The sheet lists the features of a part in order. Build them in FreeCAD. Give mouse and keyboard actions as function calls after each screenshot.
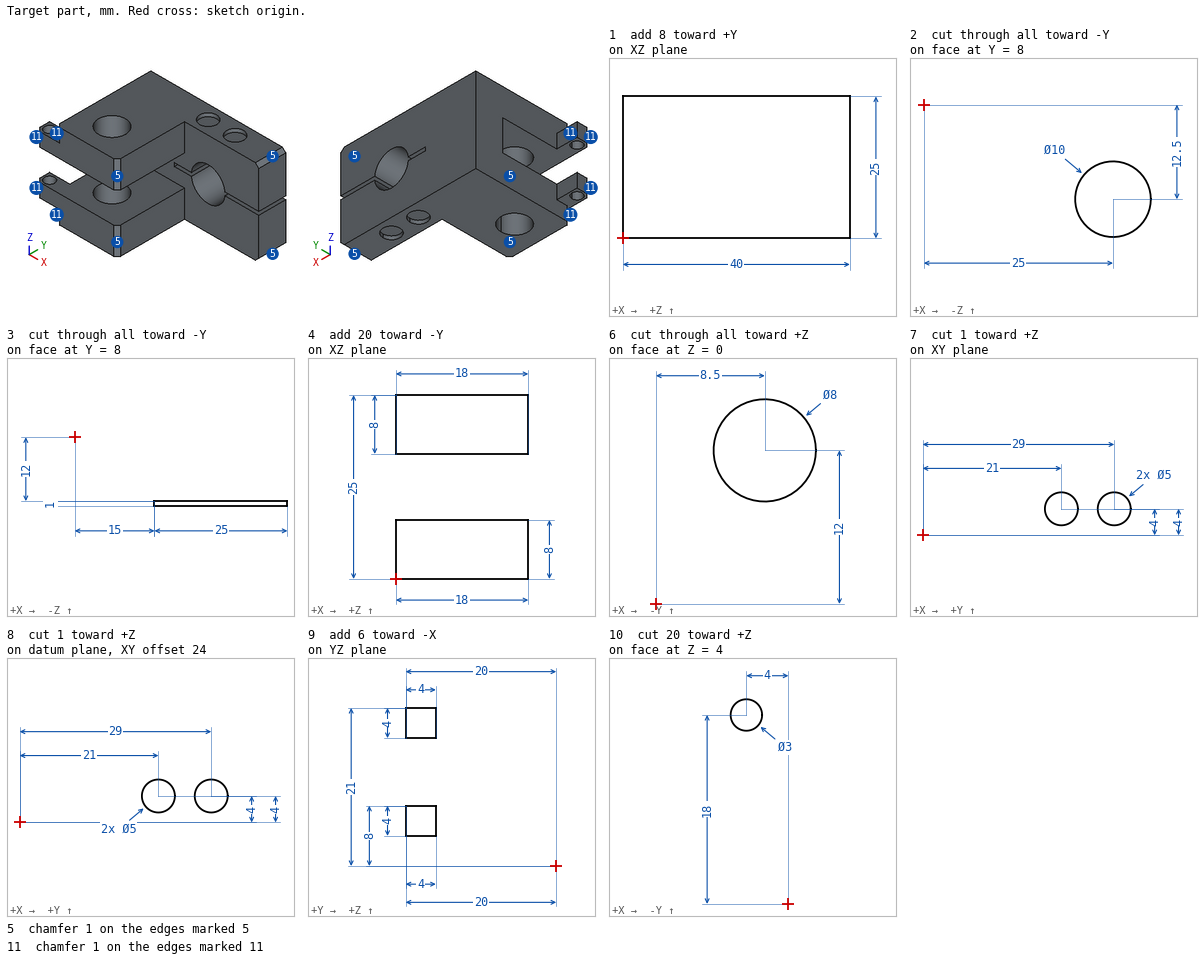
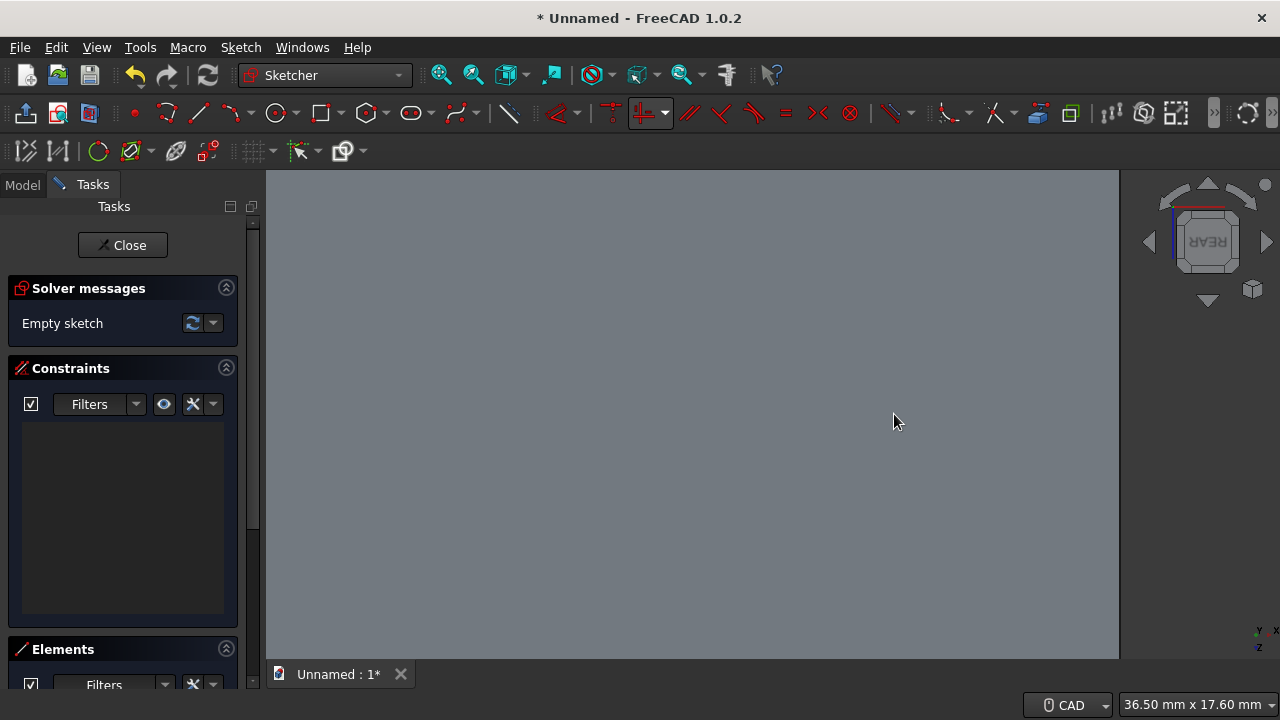
click(276, 114)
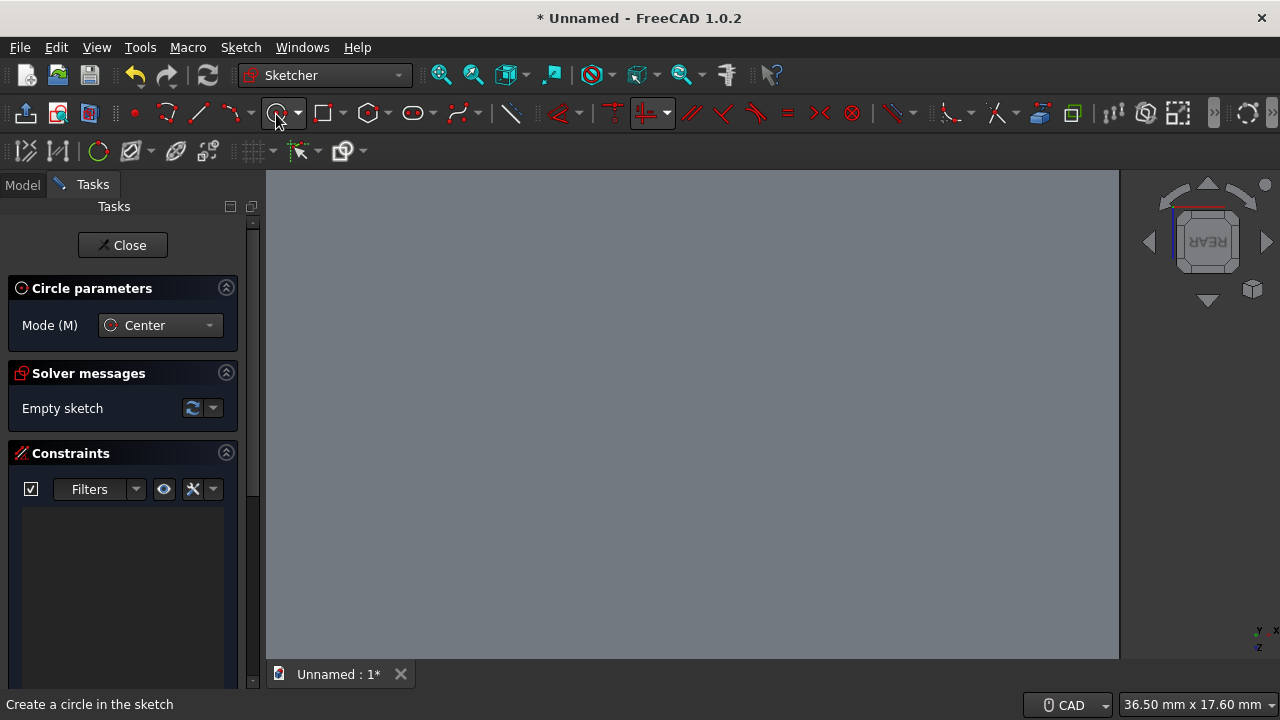
click(703, 414)
click(801, 316)
key(Escape)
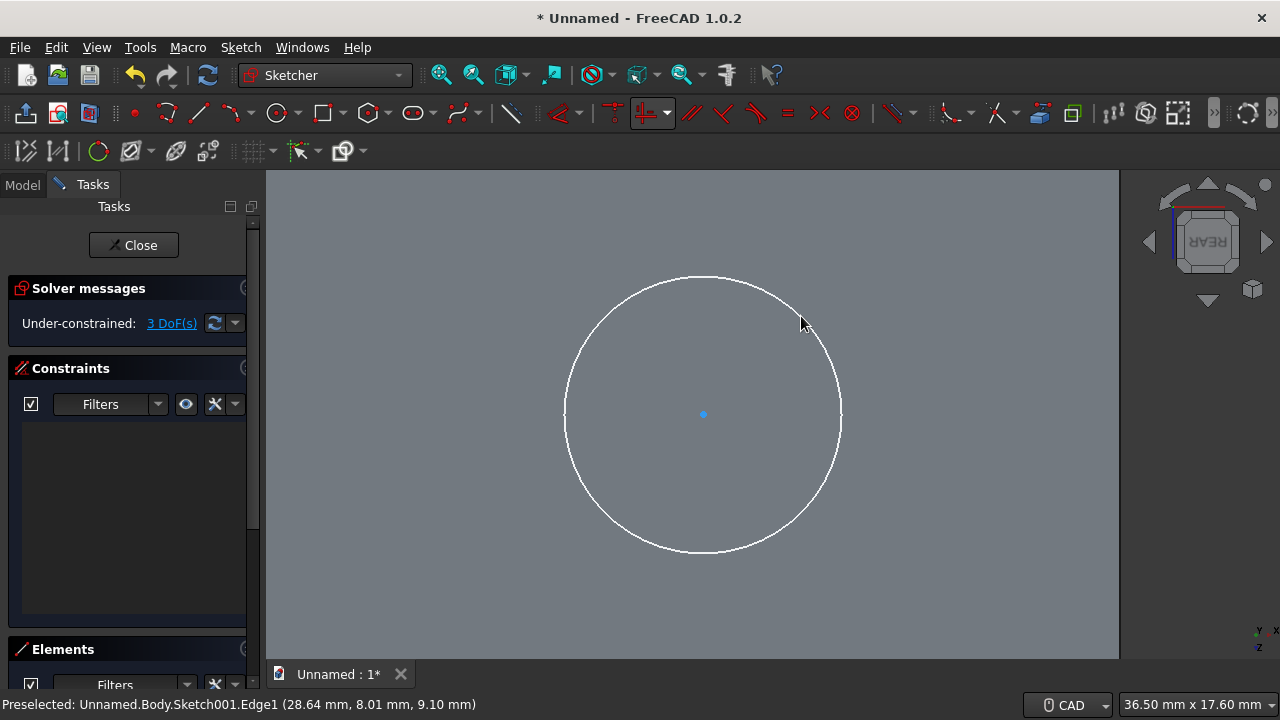
click(558, 114)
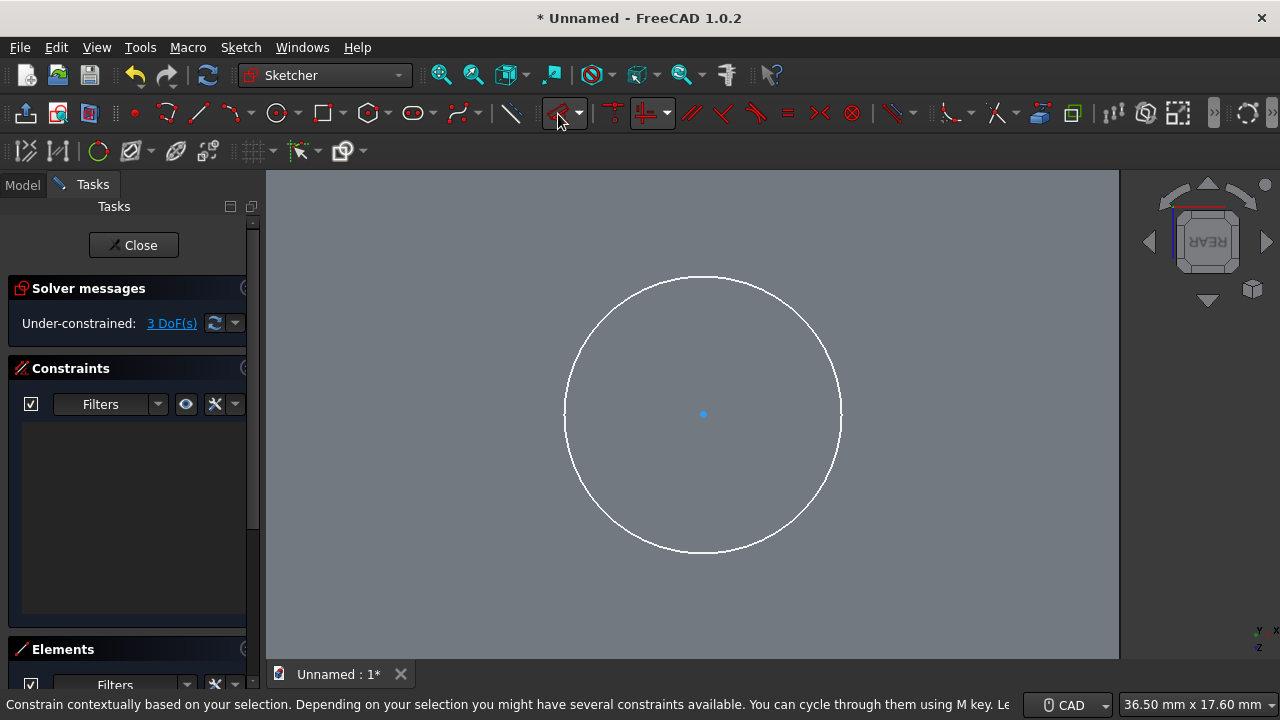
click(801, 317)
click(824, 294)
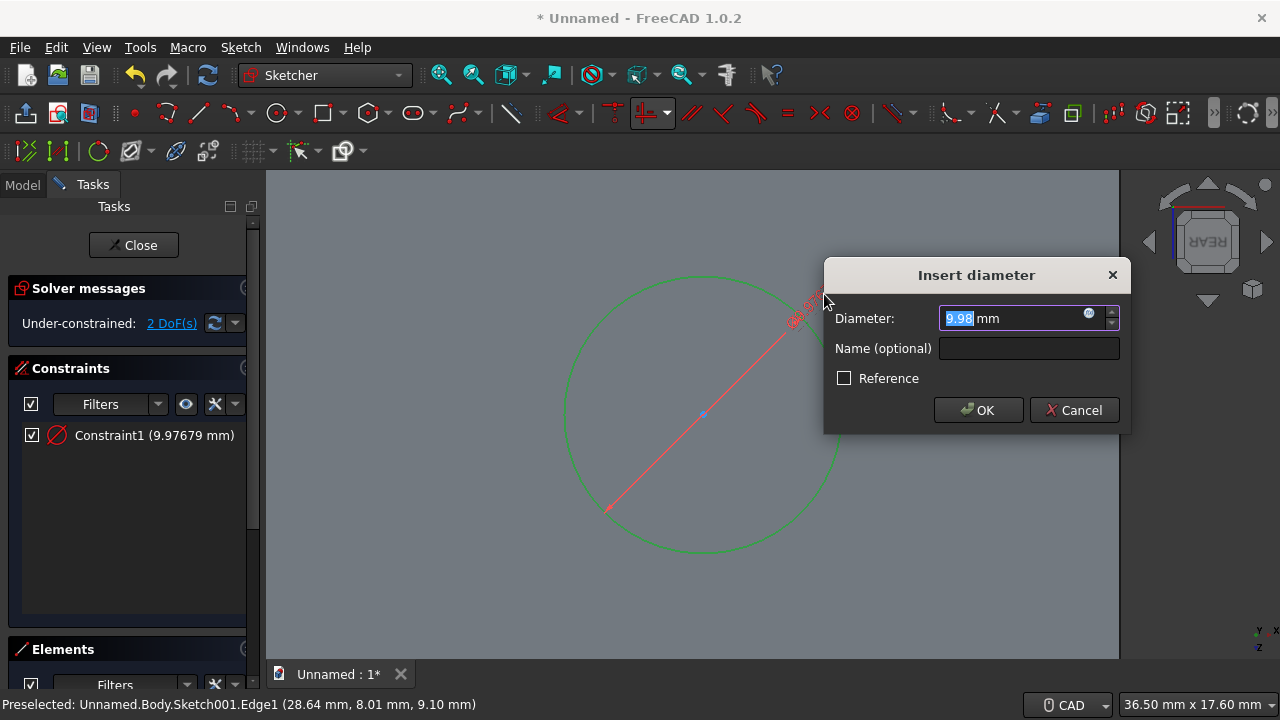
text(10)
key(Return)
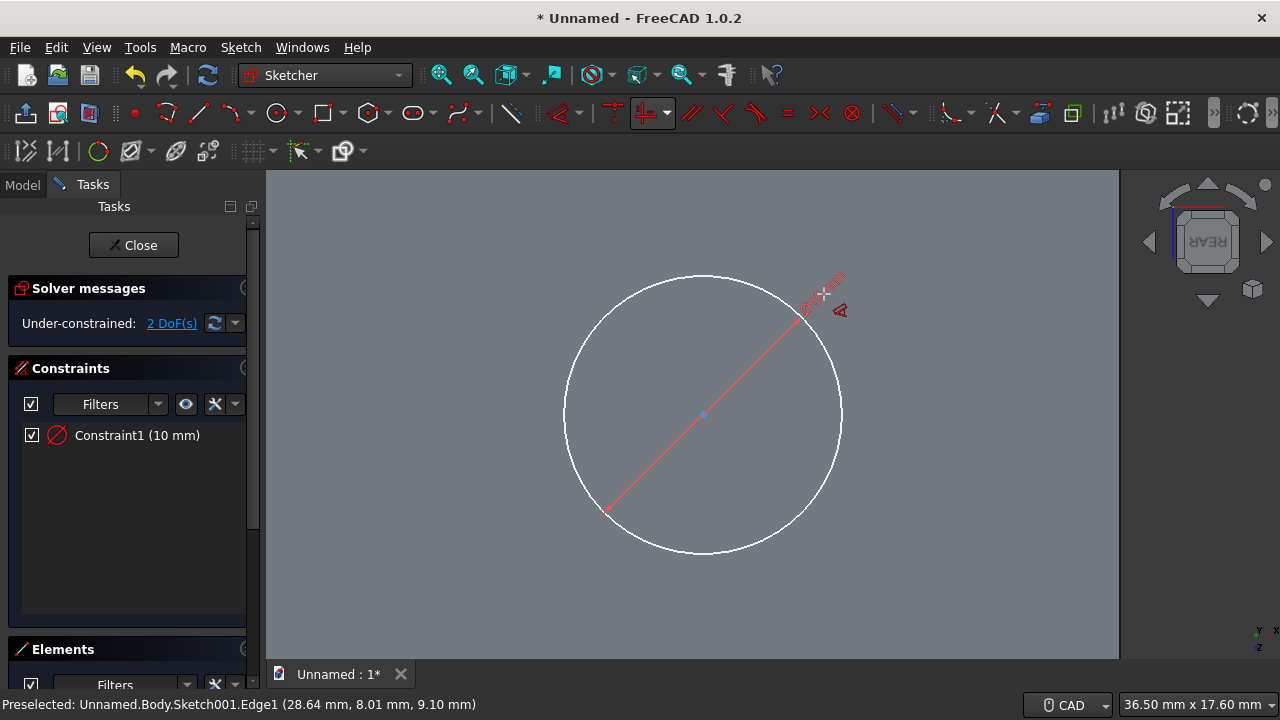
click(703, 415)
click(498, 449)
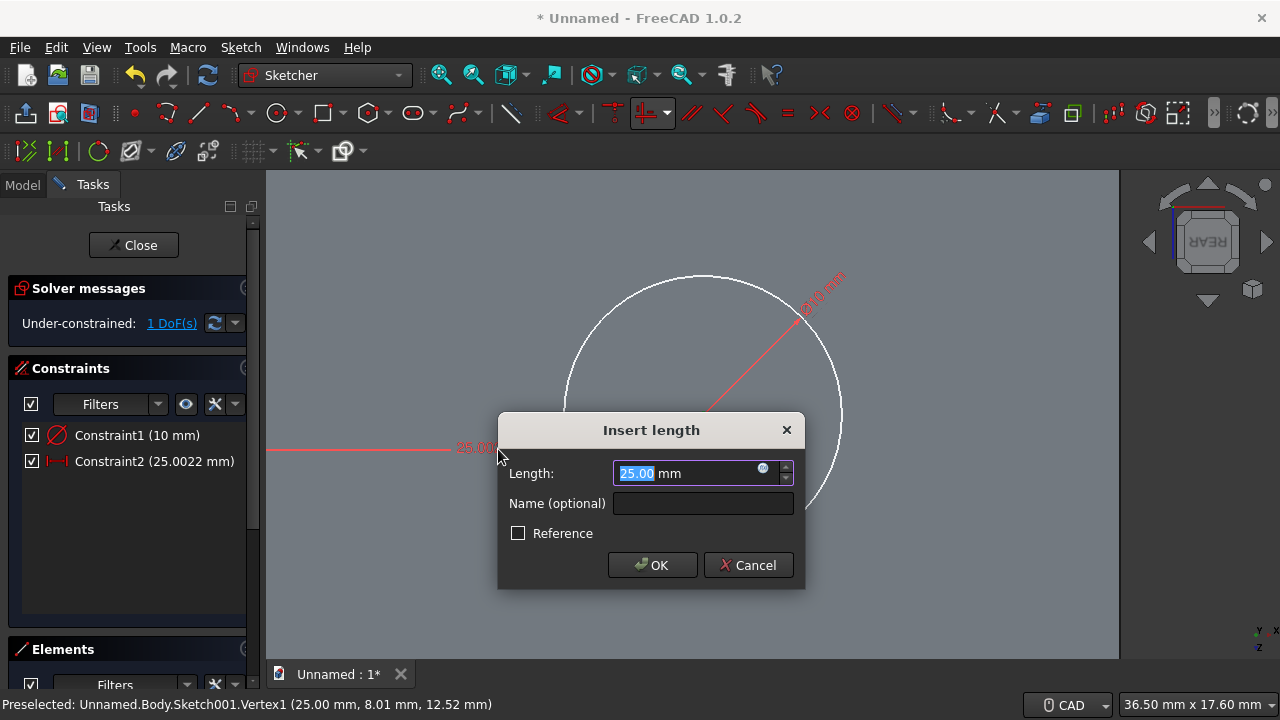
text(25)
key(Return)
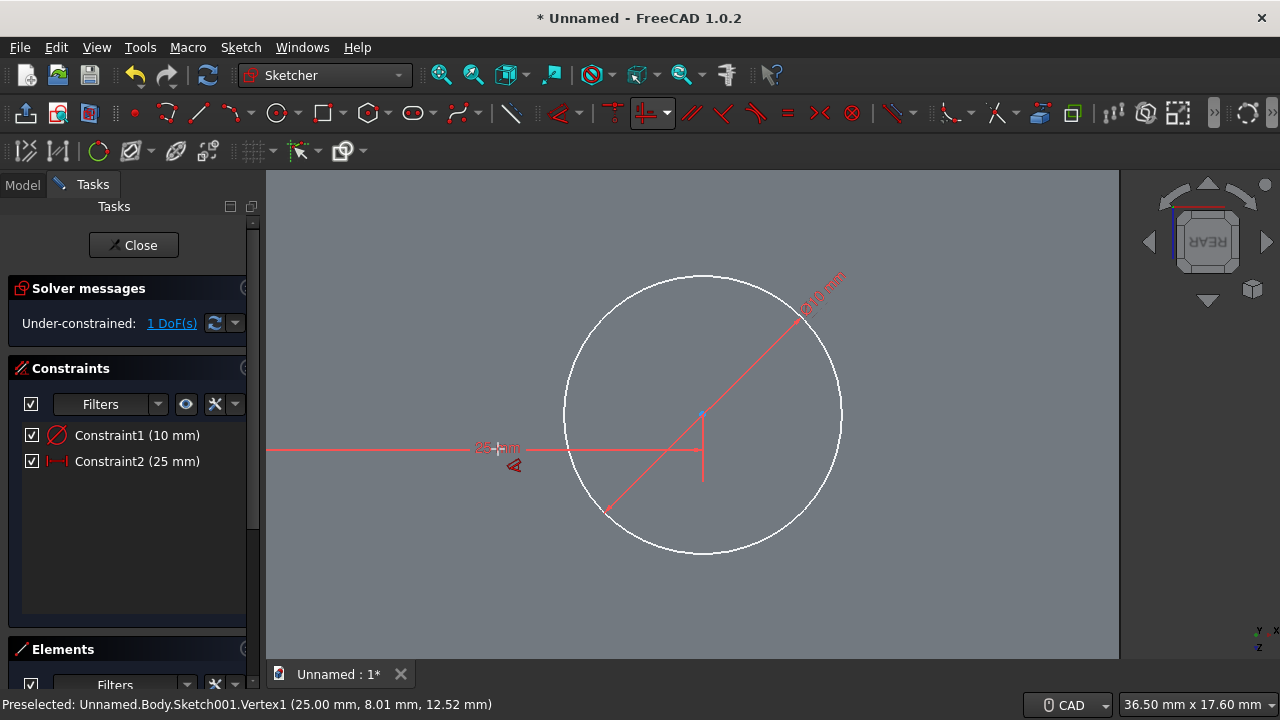
click(703, 415)
click(737, 307)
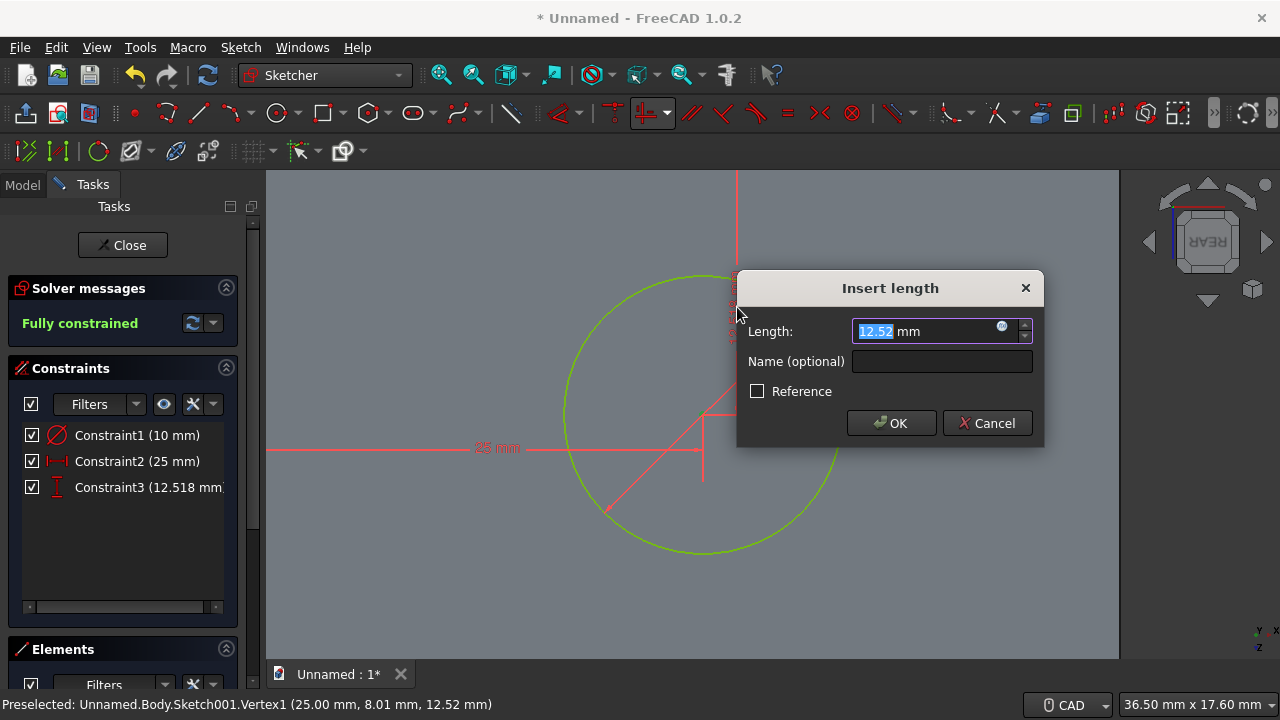
text(12.5)
key(Return)
key(Escape)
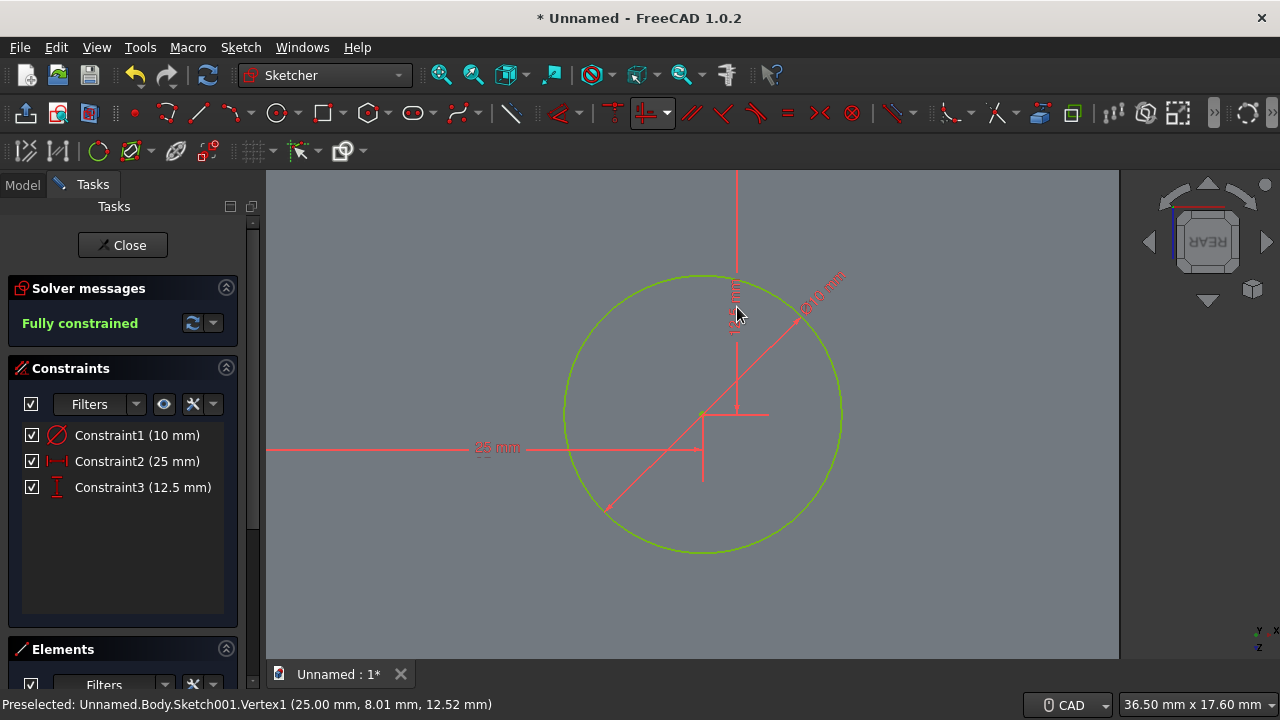
click(123, 245)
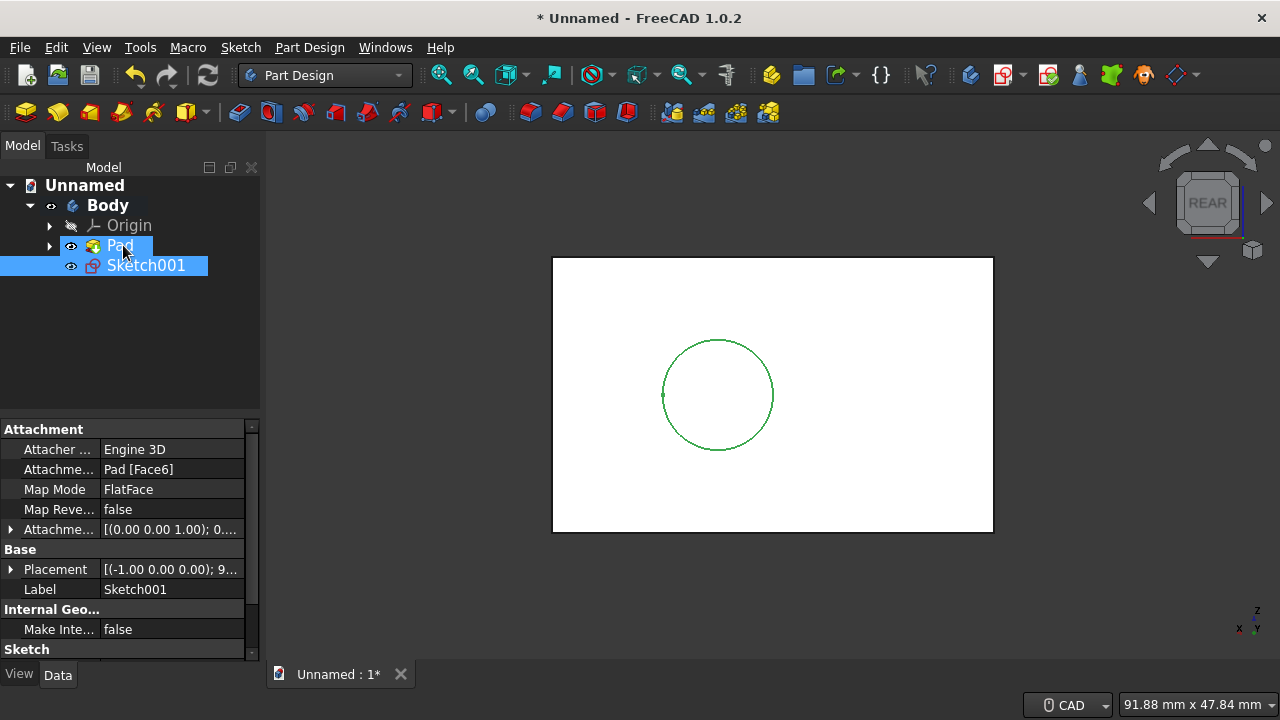
click(240, 112)